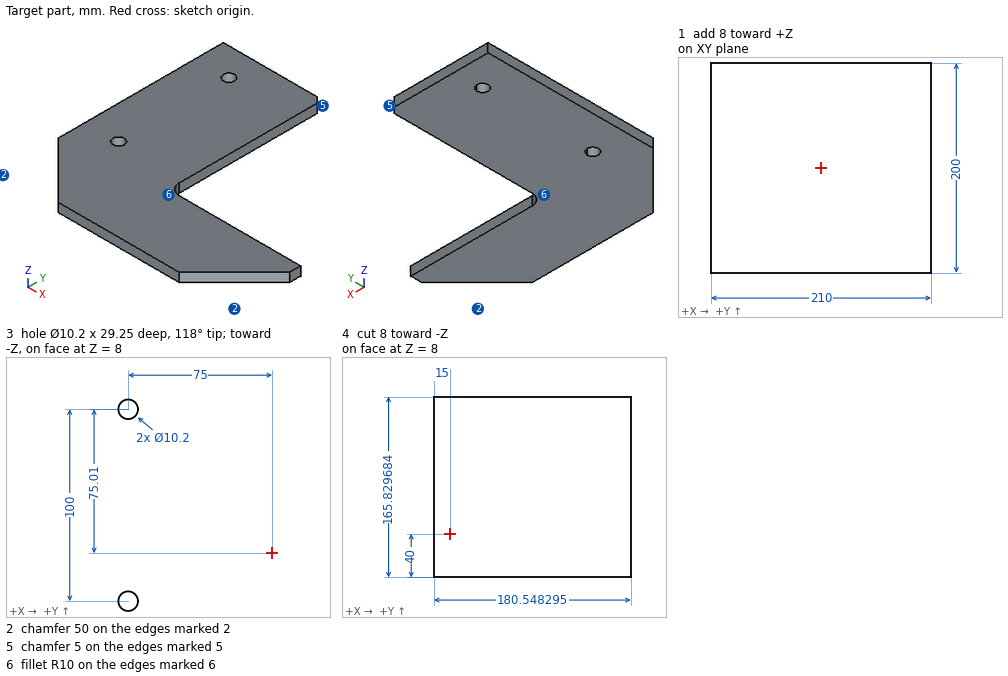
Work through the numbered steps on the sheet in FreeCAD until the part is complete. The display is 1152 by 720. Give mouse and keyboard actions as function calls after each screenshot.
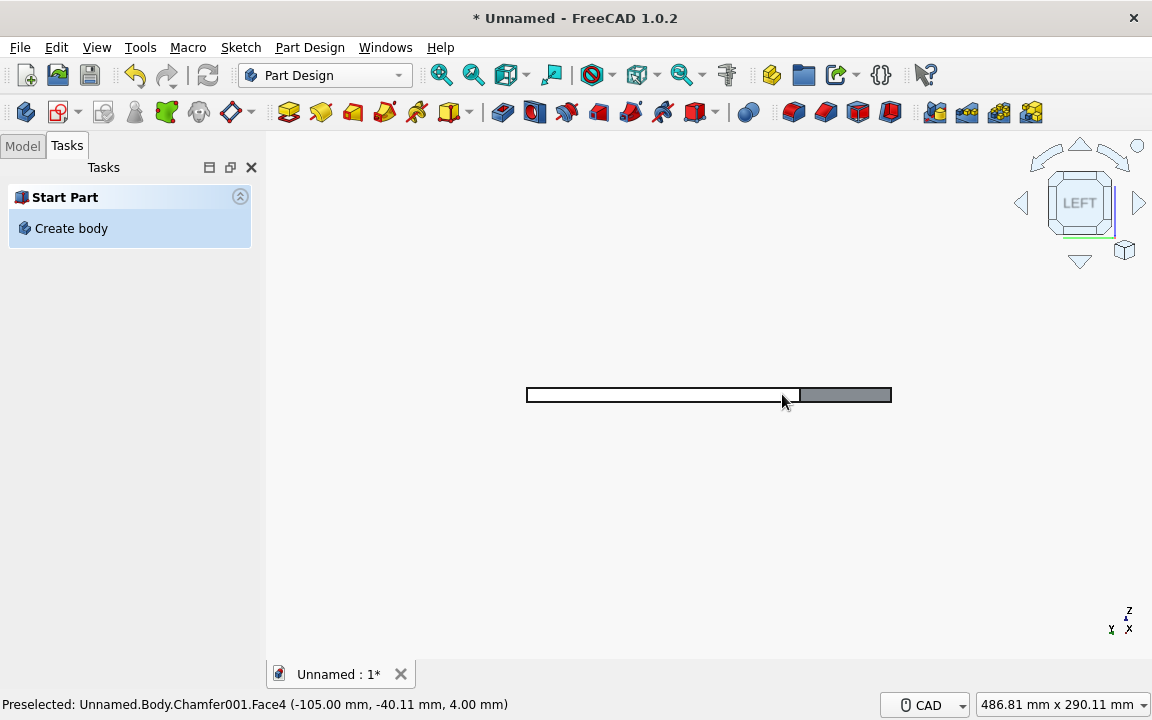
key(v)
key(3)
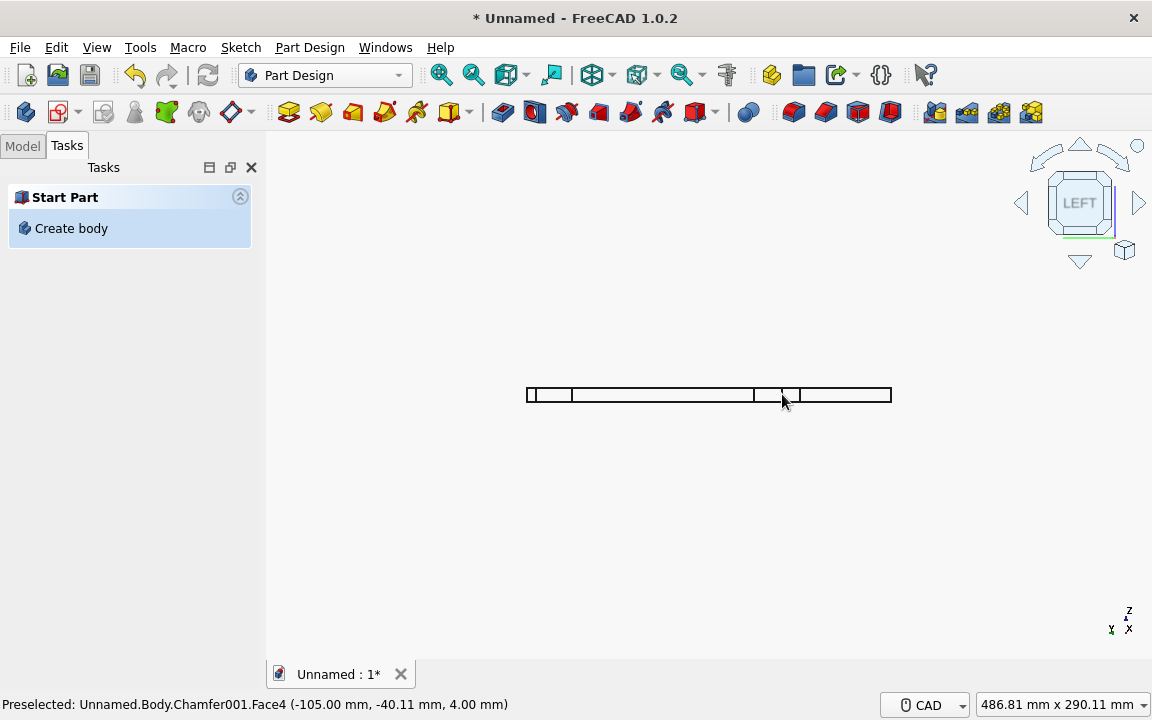
key(0)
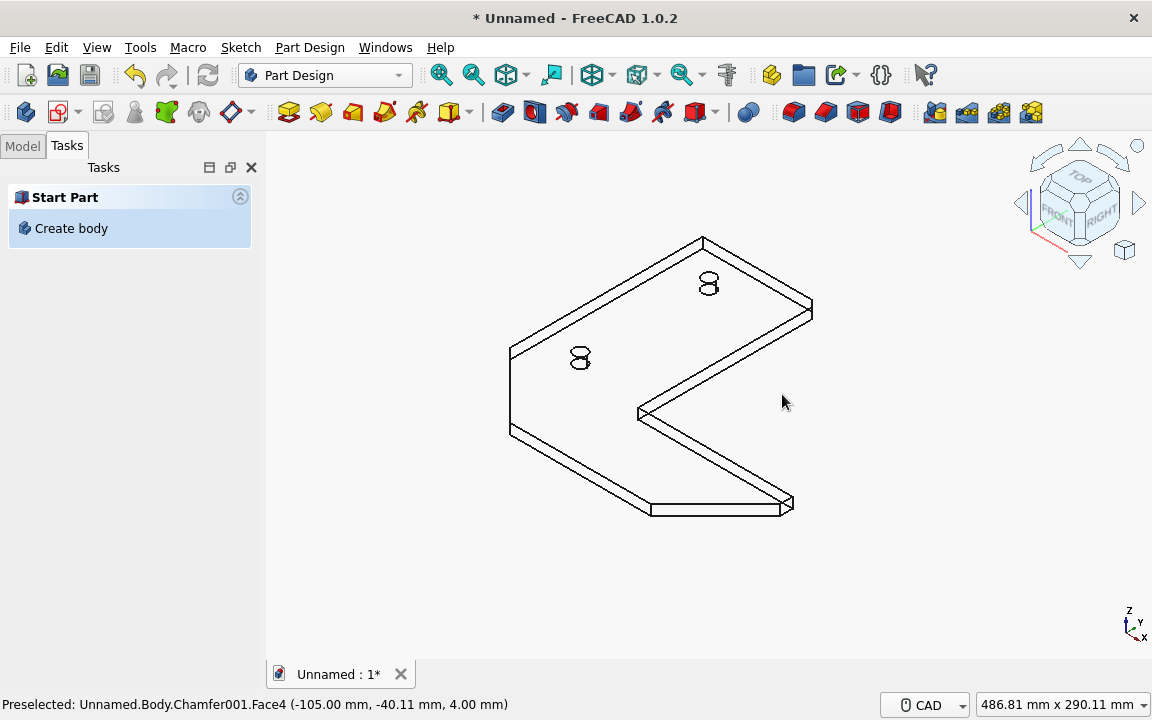
click(638, 414)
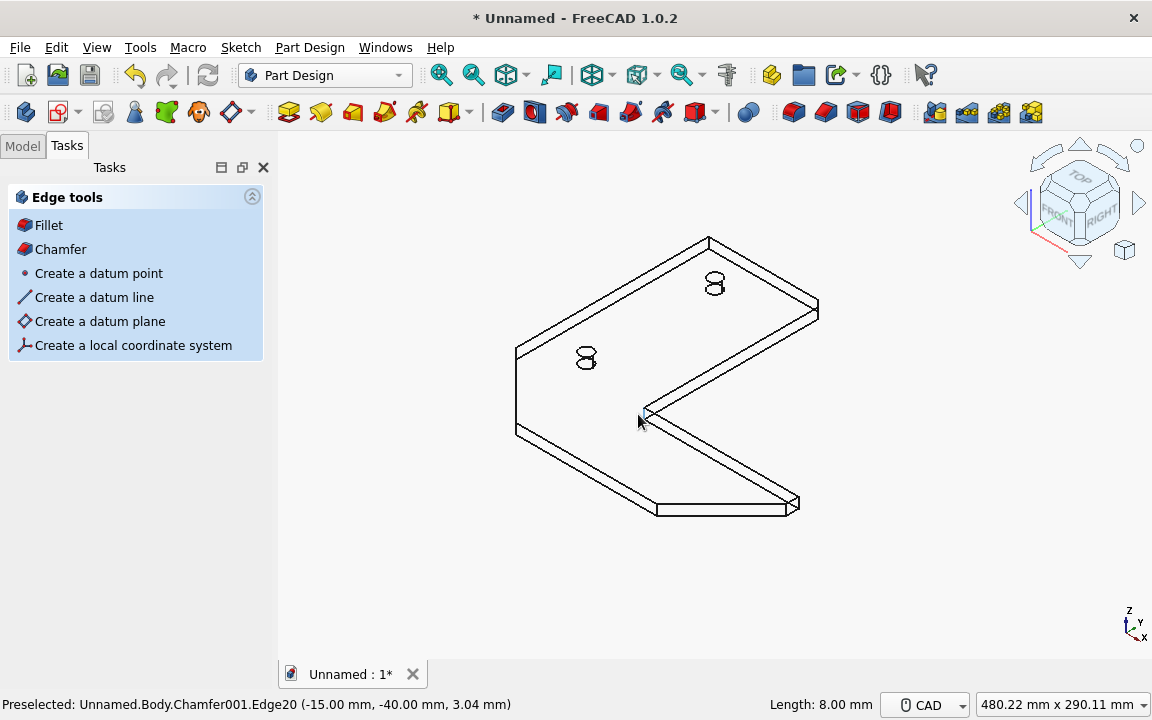
key(v)
key(1)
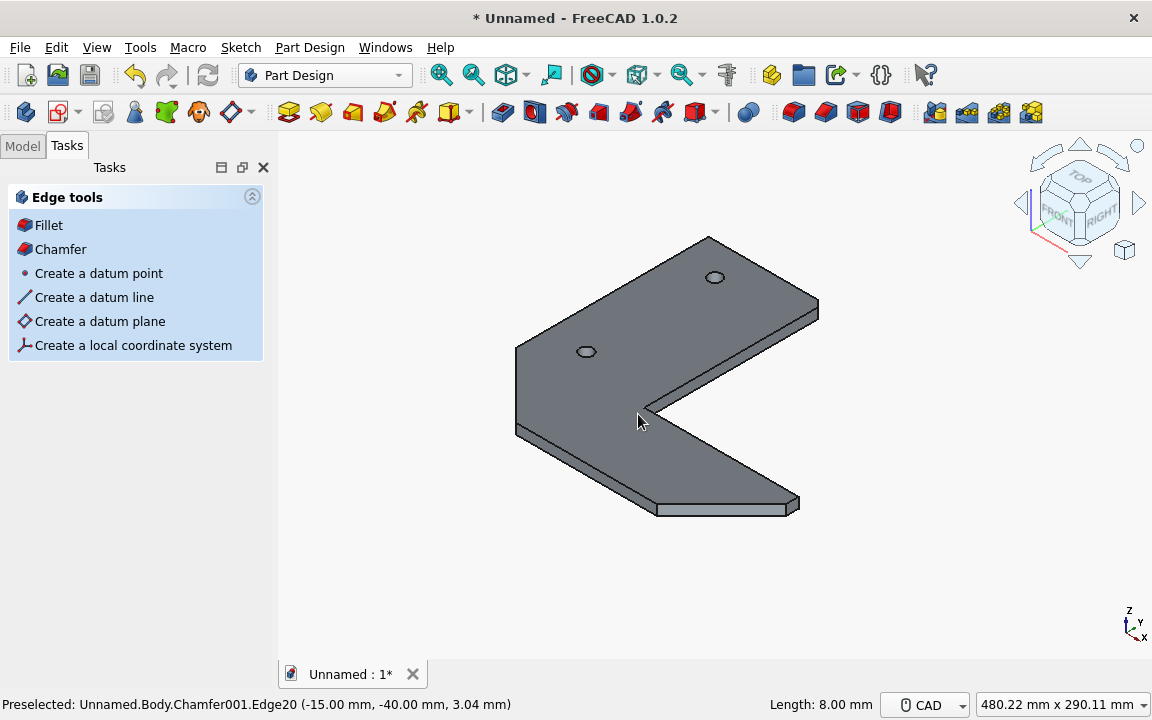
click(794, 112)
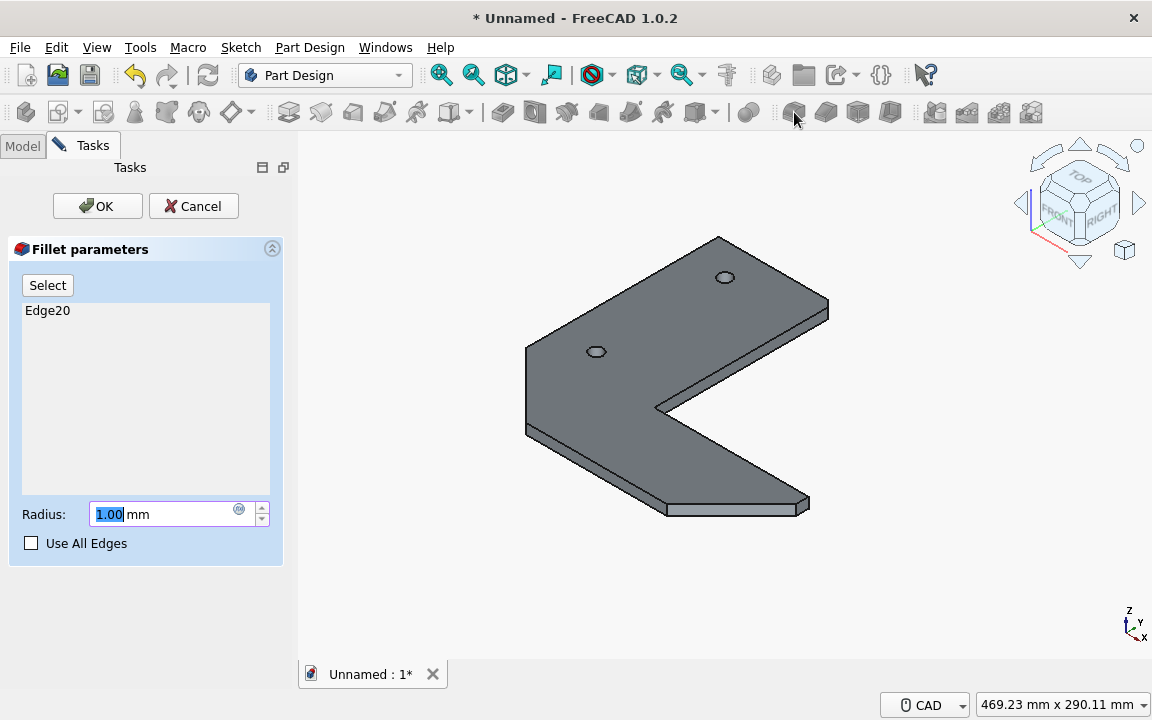
text(10)
key(Tab)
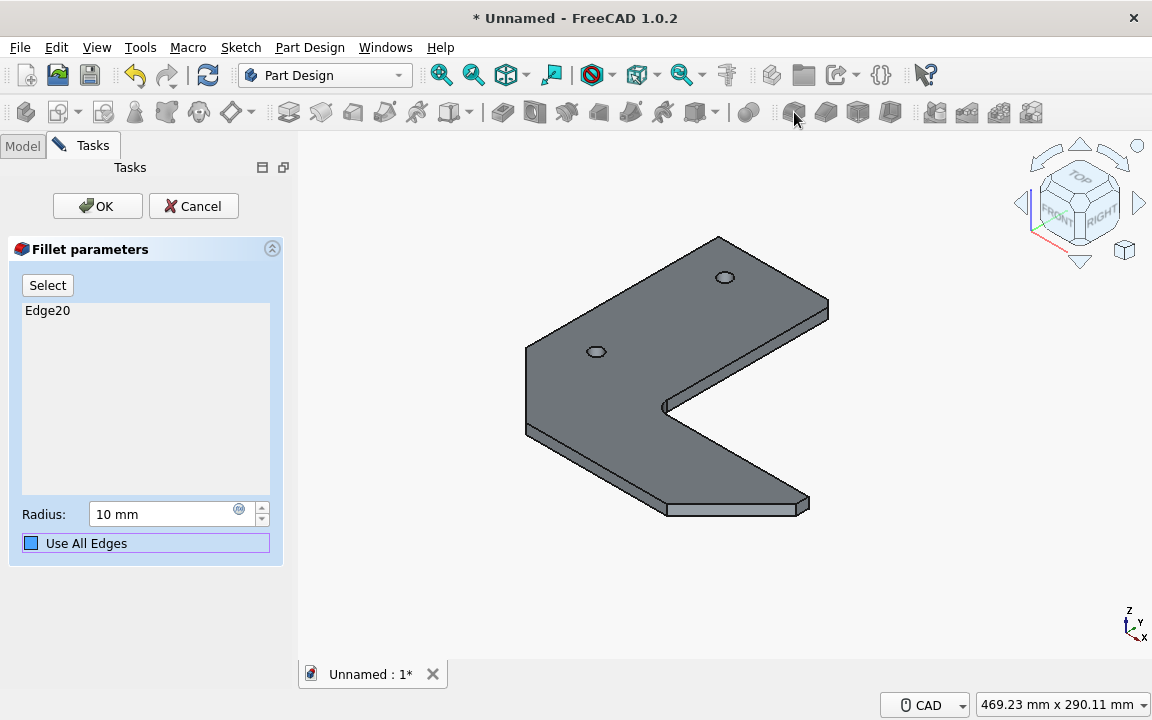
click(98, 206)